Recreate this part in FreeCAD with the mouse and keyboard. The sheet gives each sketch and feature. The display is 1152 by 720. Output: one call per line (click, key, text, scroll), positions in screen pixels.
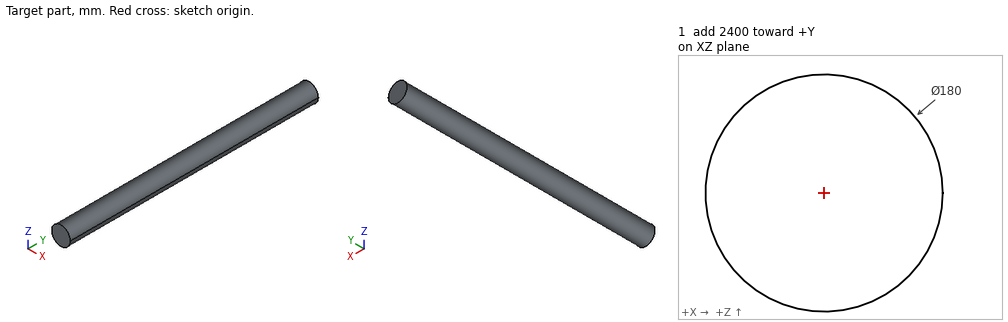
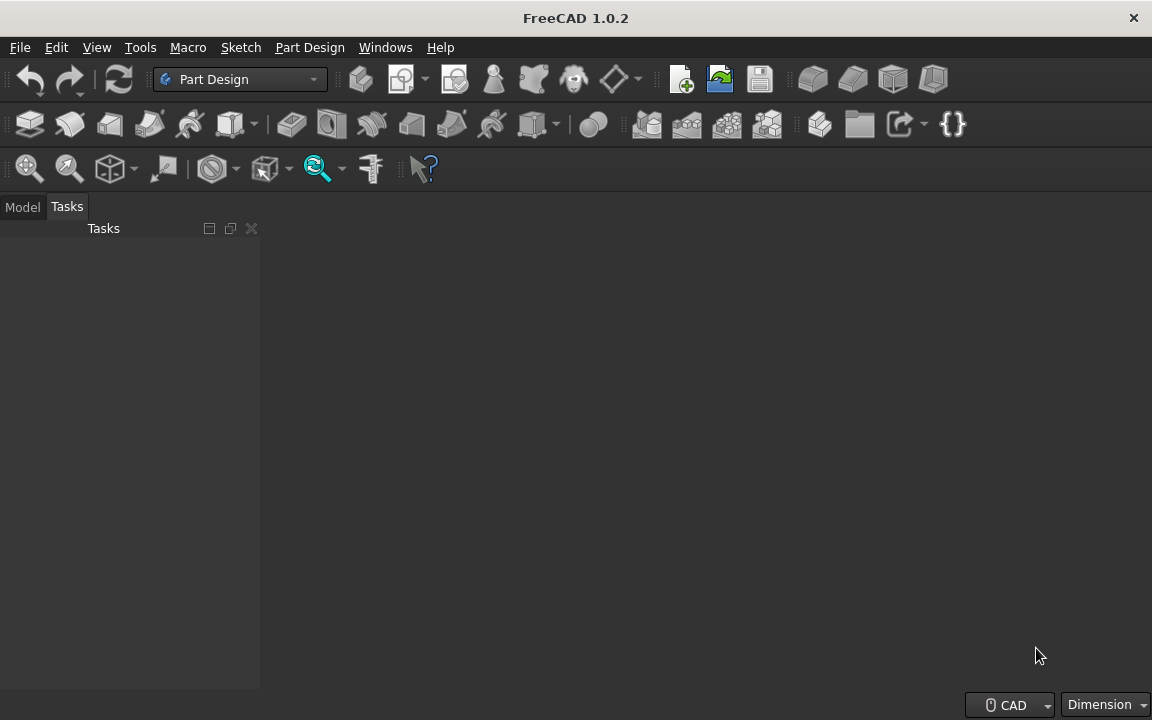
key(ctrl+n)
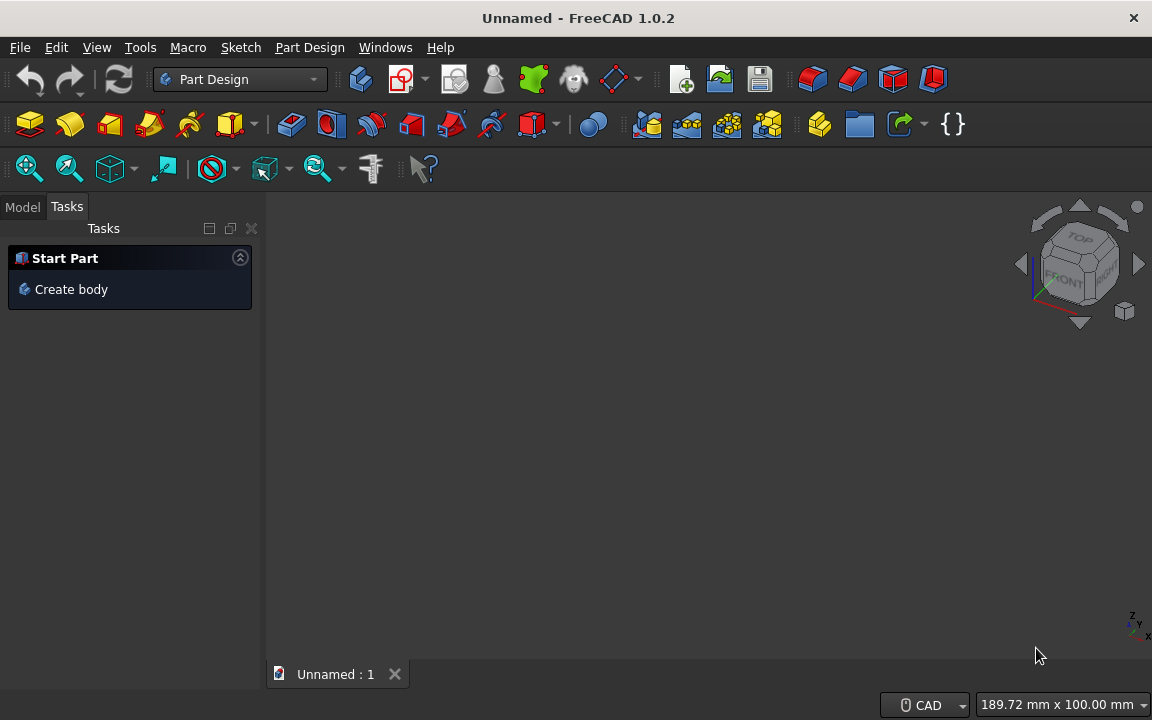
click(402, 80)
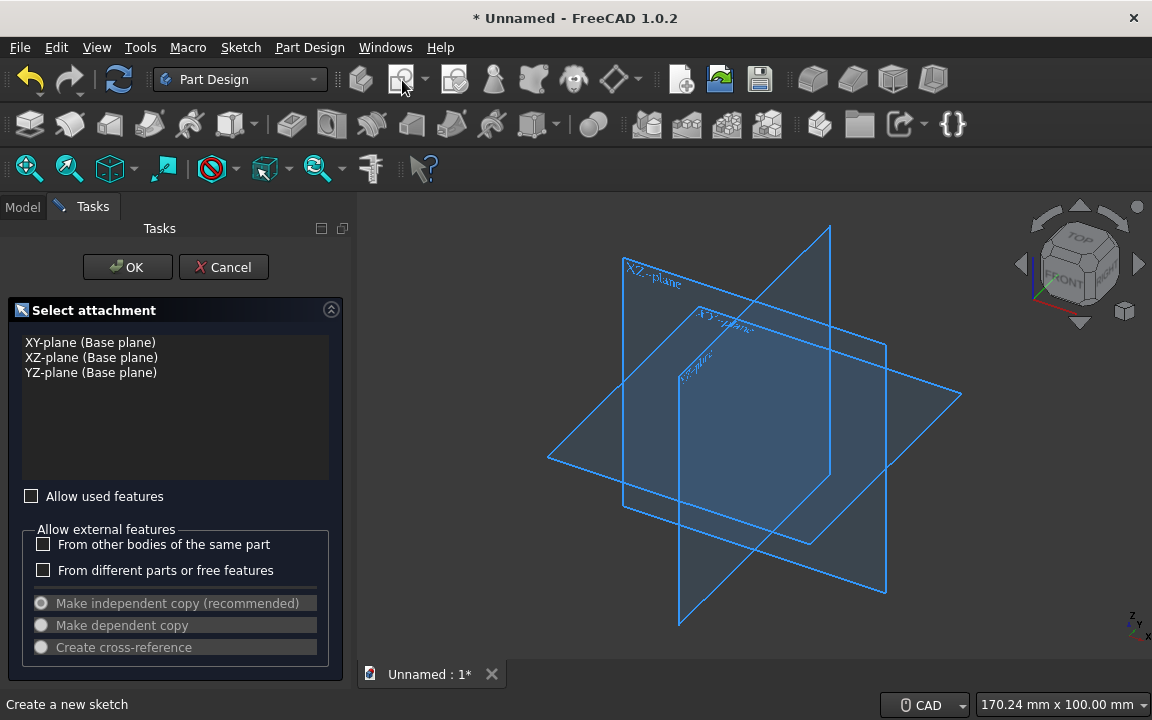
click(82, 358)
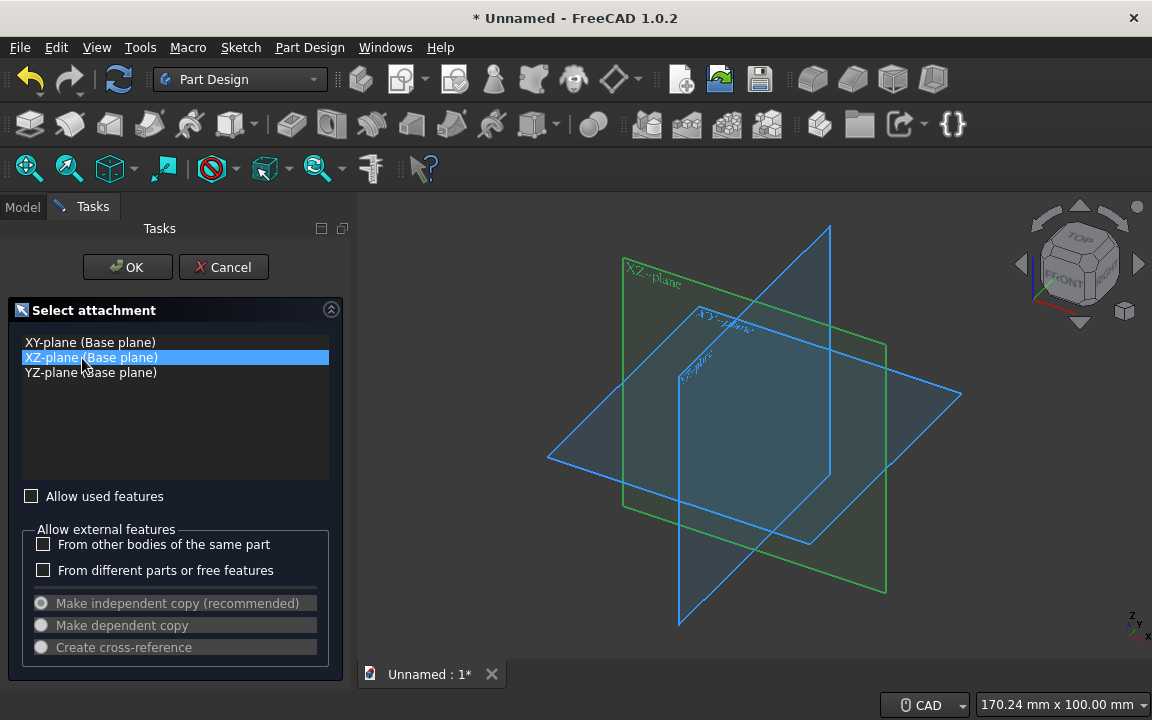
click(128, 267)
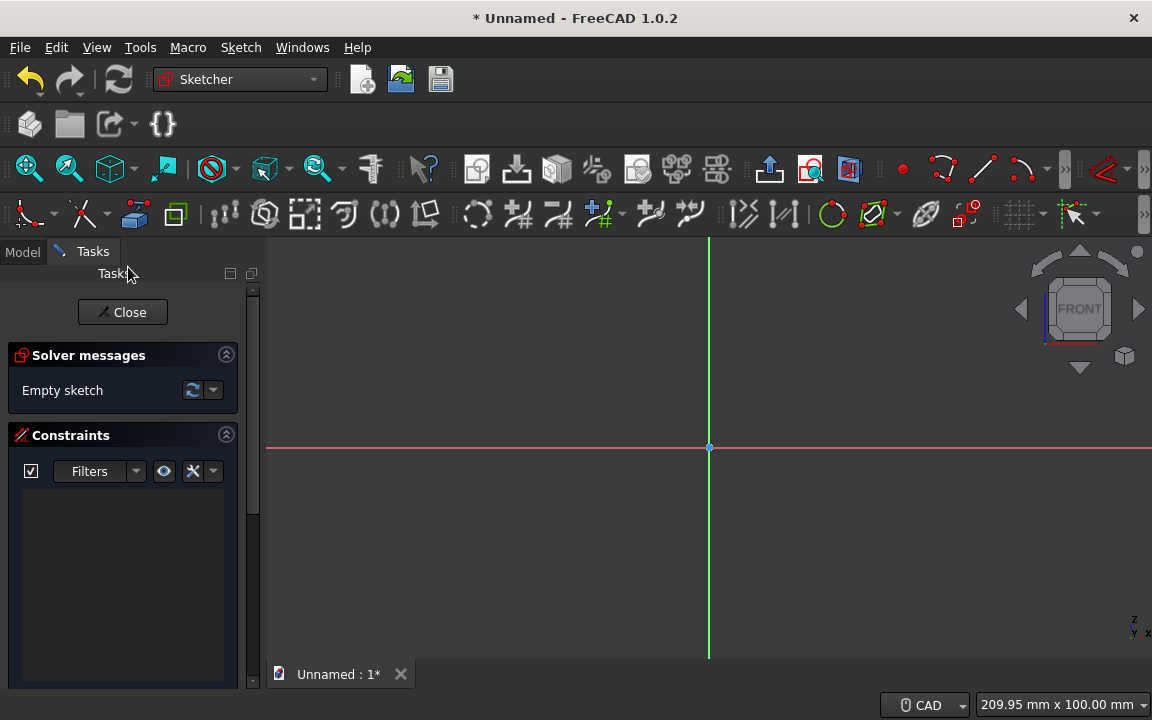
scroll(601, 448, down, 5)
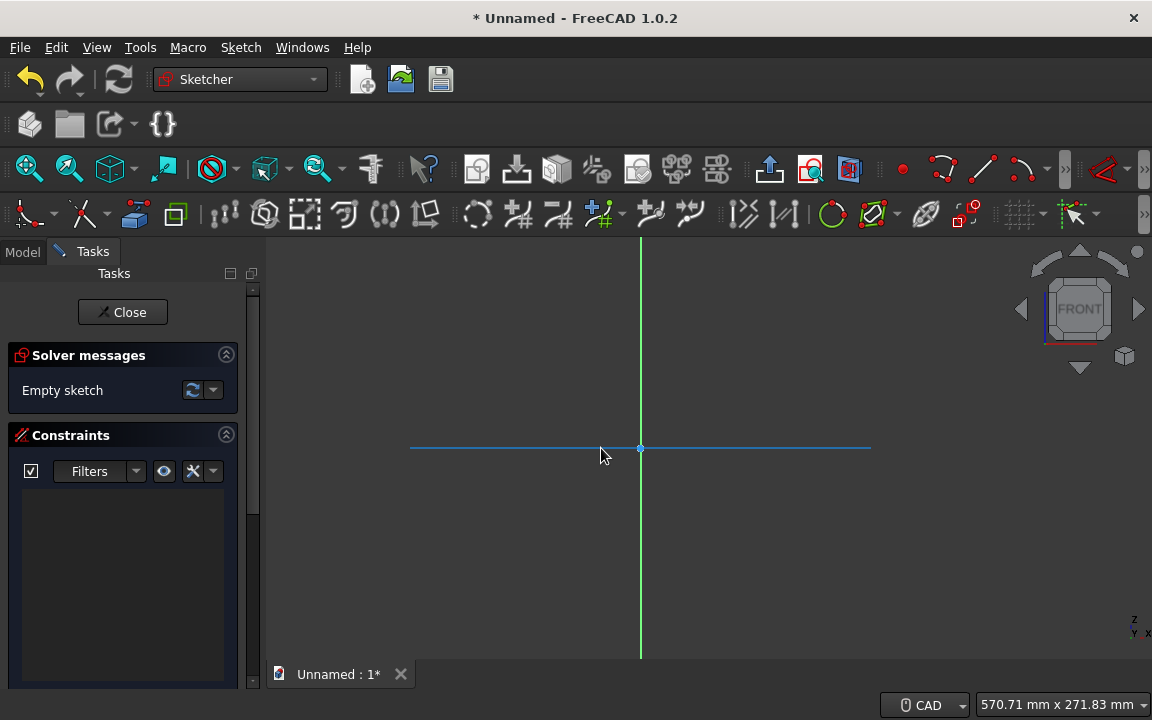
key(g)
key(c)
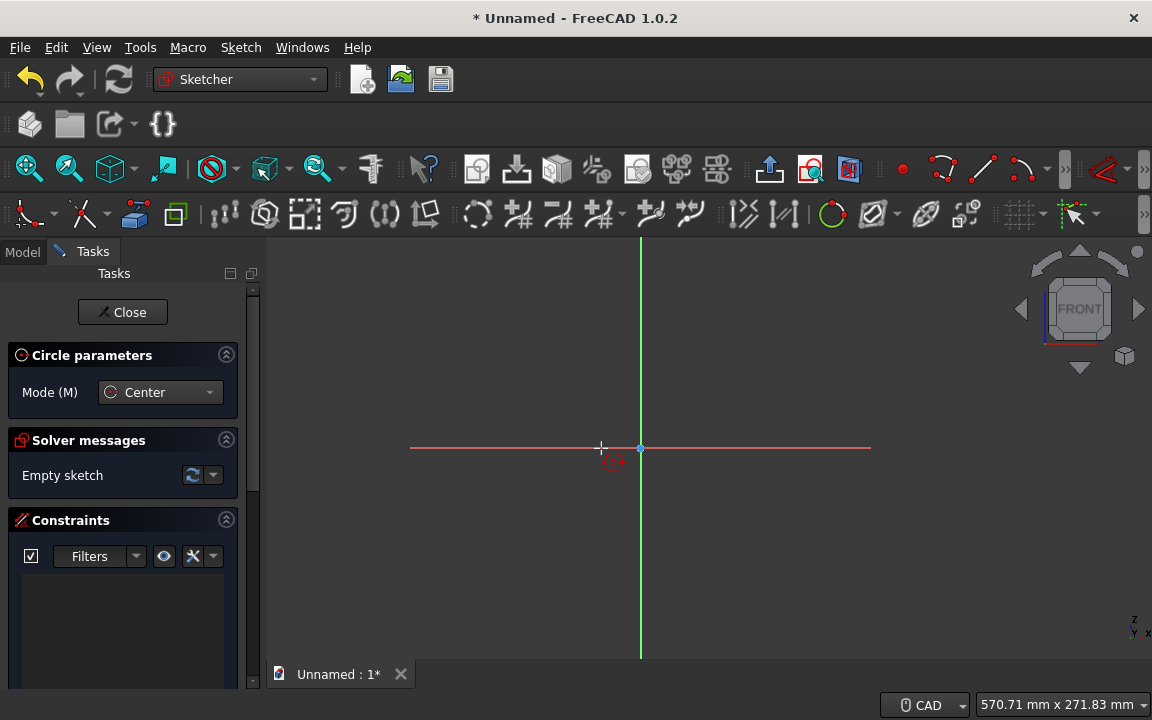
click(641, 448)
click(740, 350)
key(Escape)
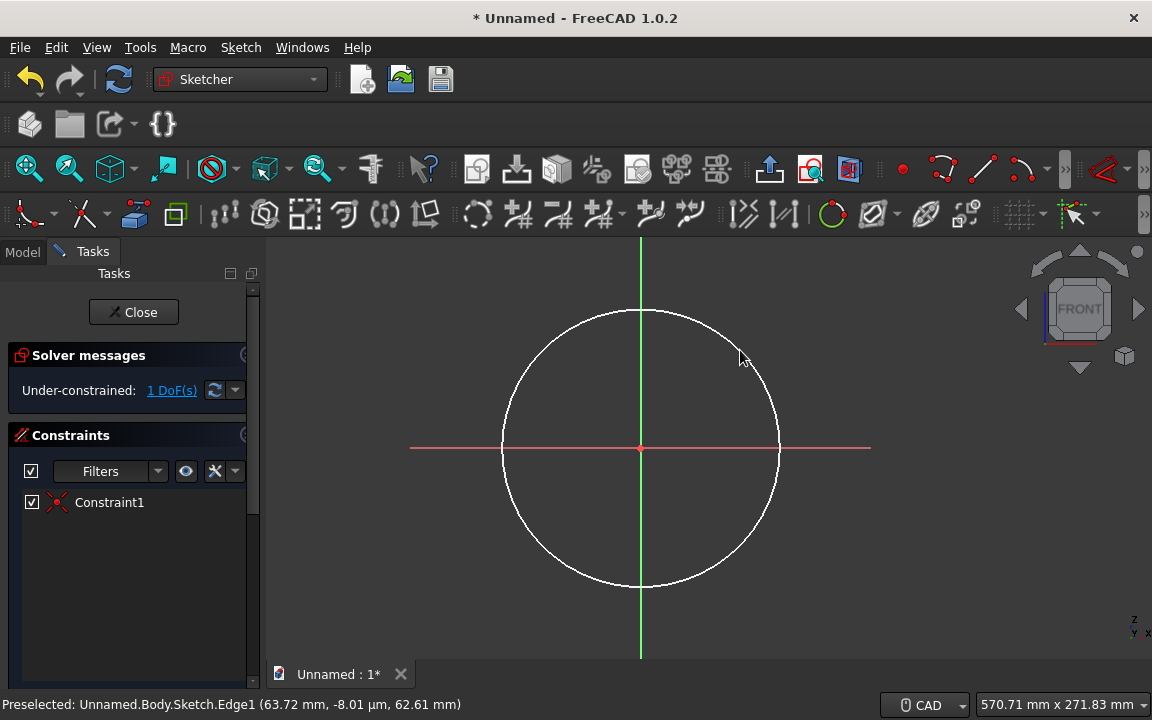
click(1104, 170)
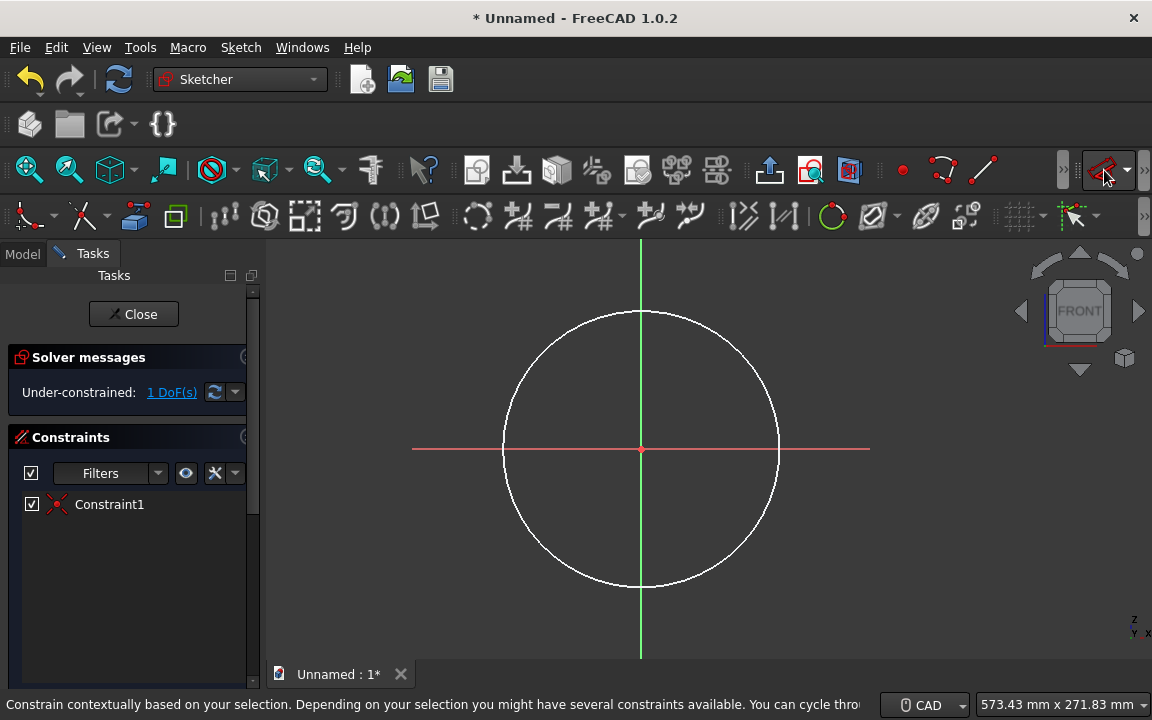
click(739, 351)
click(762, 328)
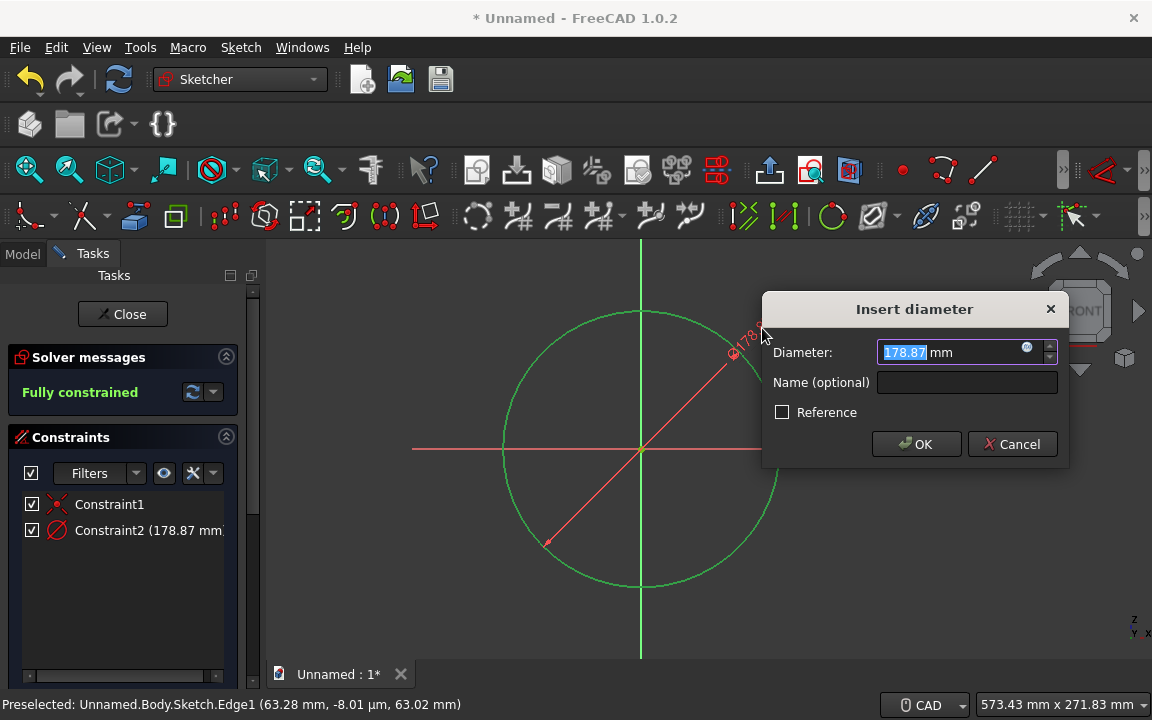
text(180)
key(Return)
key(Escape)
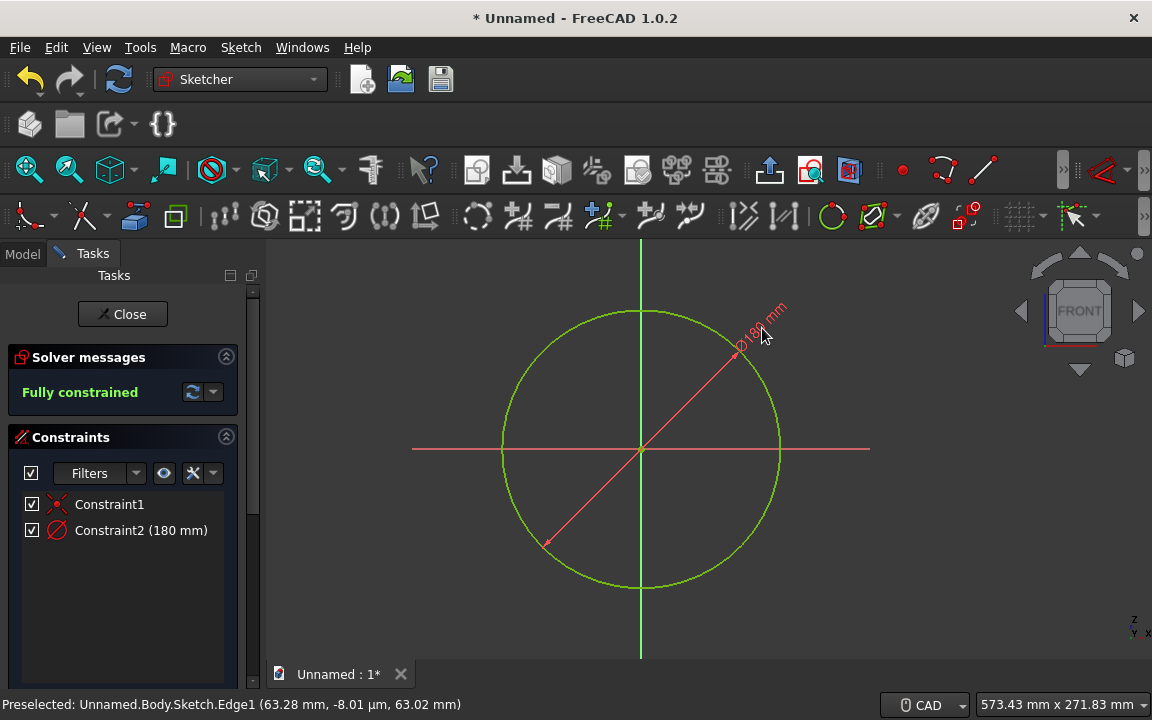
click(123, 314)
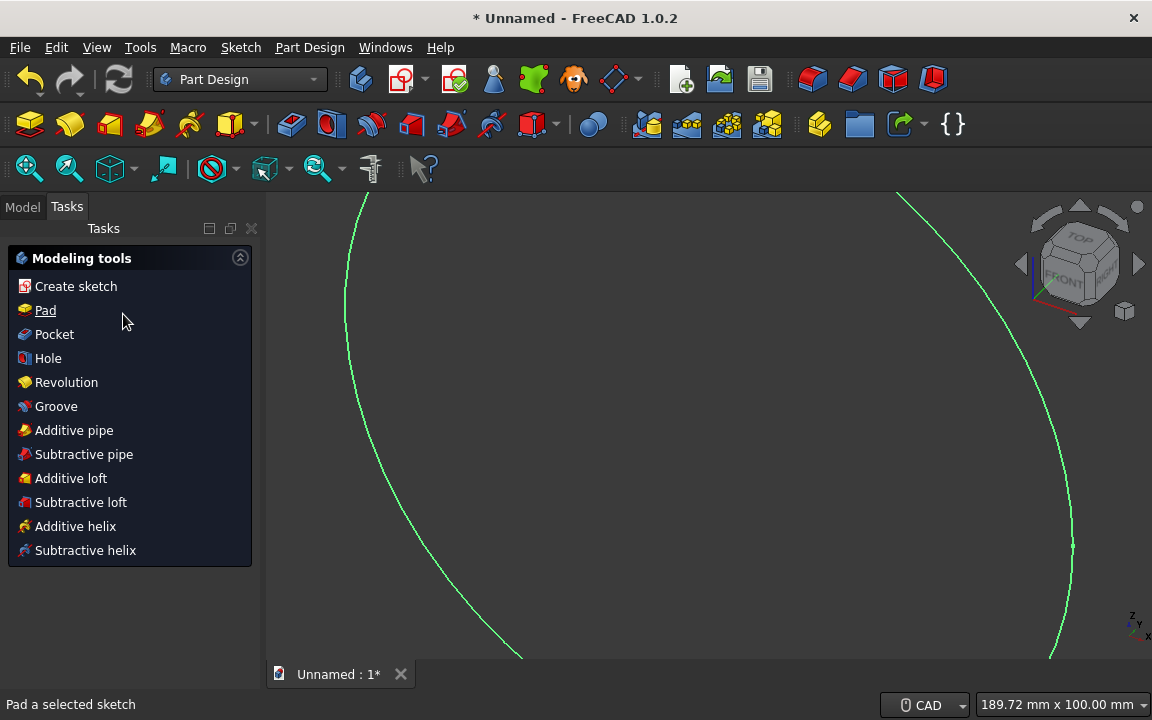
click(30, 124)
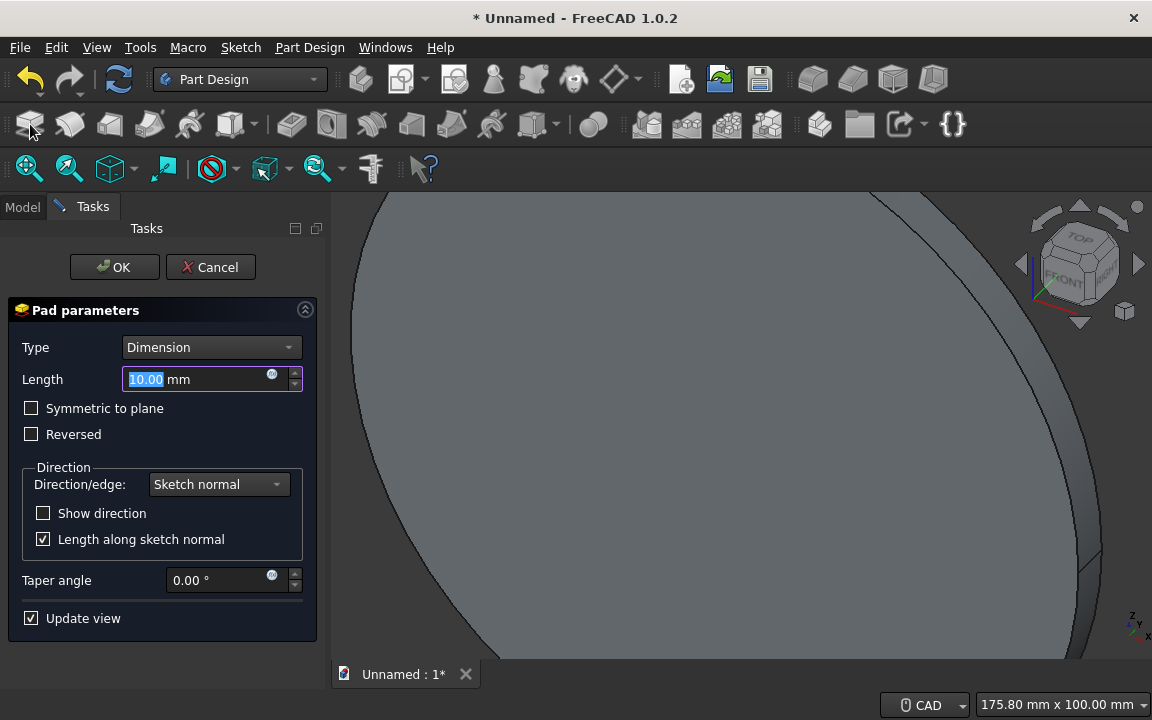
text(2400)
key(Tab)